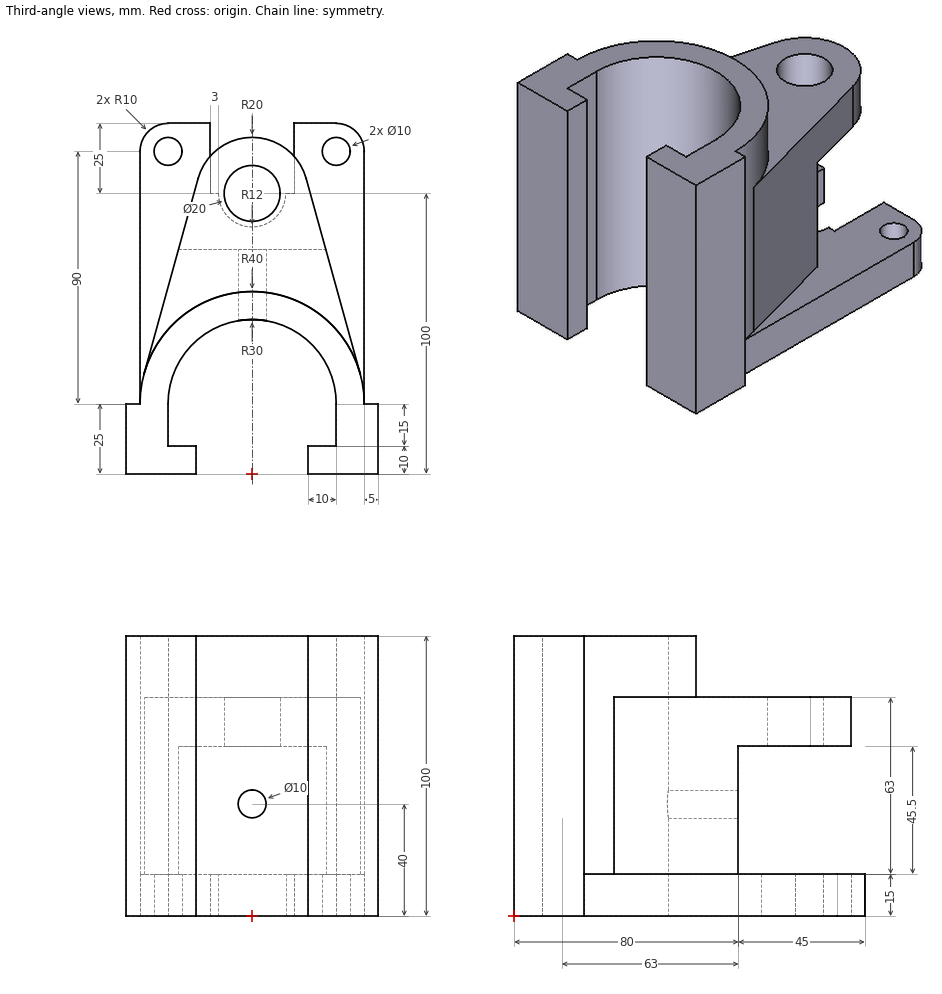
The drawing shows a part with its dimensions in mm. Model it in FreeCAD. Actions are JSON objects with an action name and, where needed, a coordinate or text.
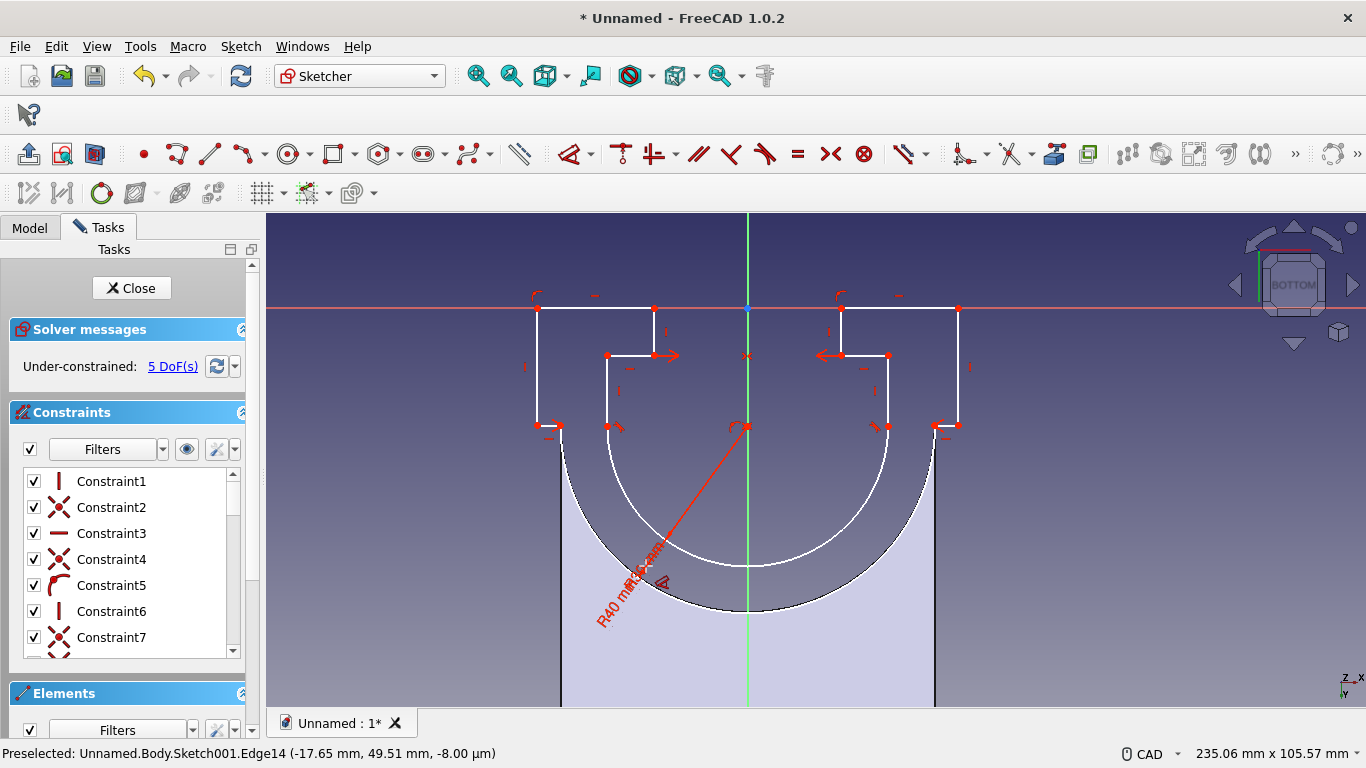
{"action": "scroll", "coordinate": [949, 426], "scroll_direction": "up", "scroll_amount": 3}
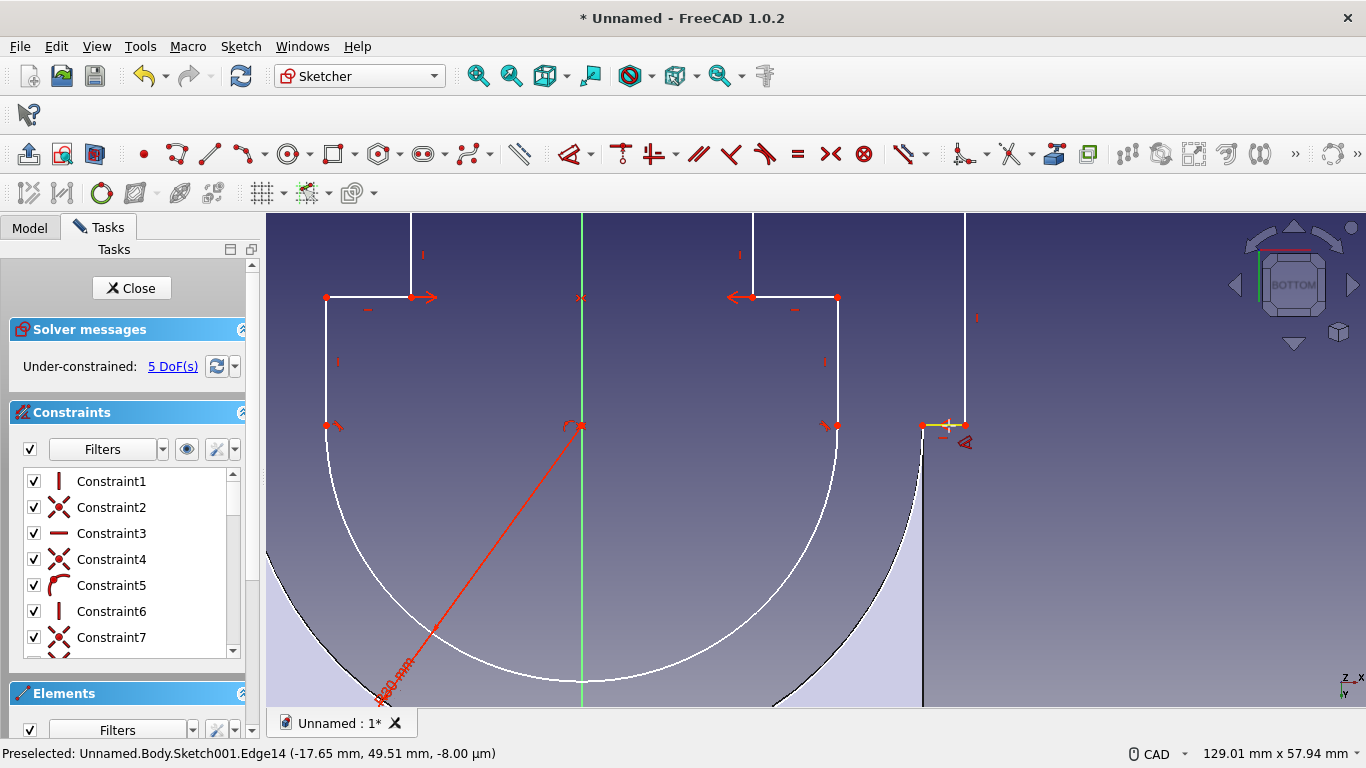
{"action": "left_click", "coordinate": [948, 425]}
{"action": "left_click", "coordinate": [944, 391]}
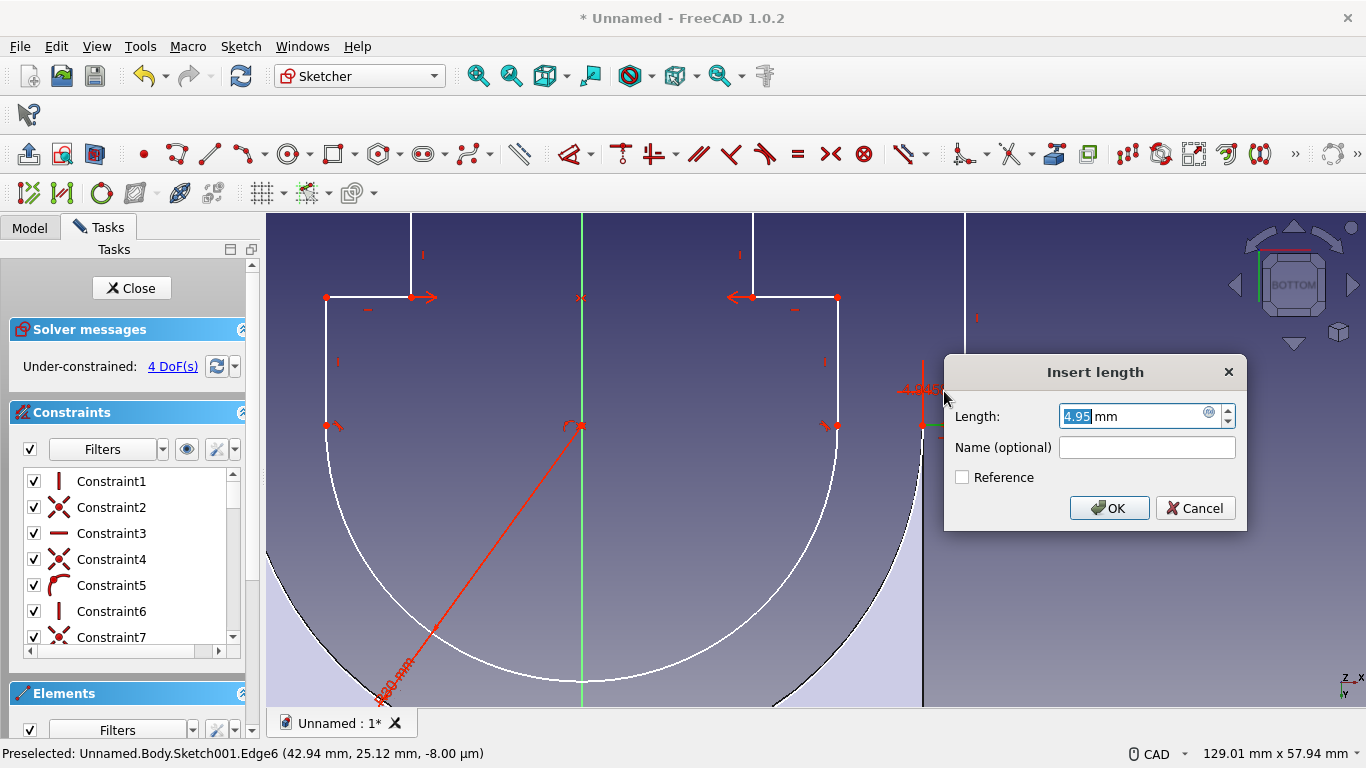
{"action": "type", "text": "5"}
{"action": "key", "text": "Return"}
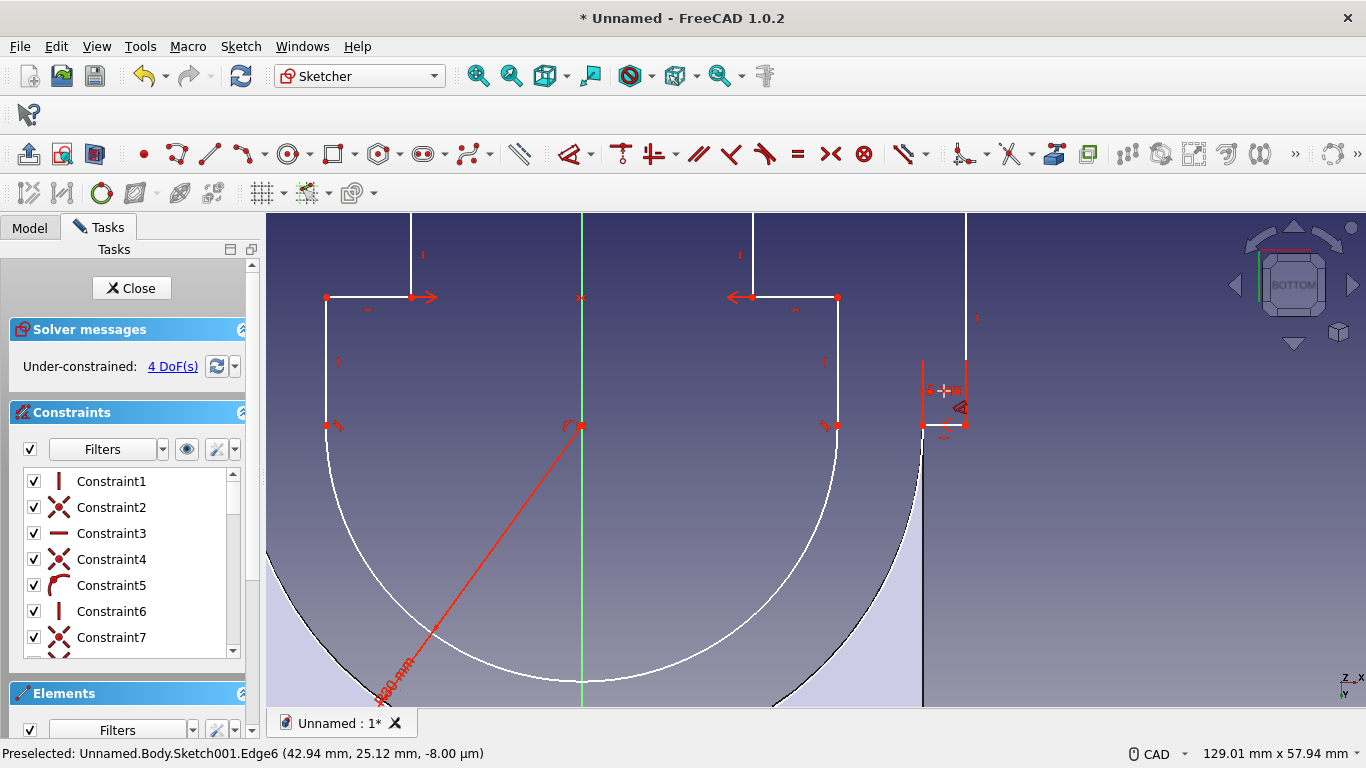
{"action": "left_click", "coordinate": [838, 387]}
{"action": "left_click", "coordinate": [872, 362]}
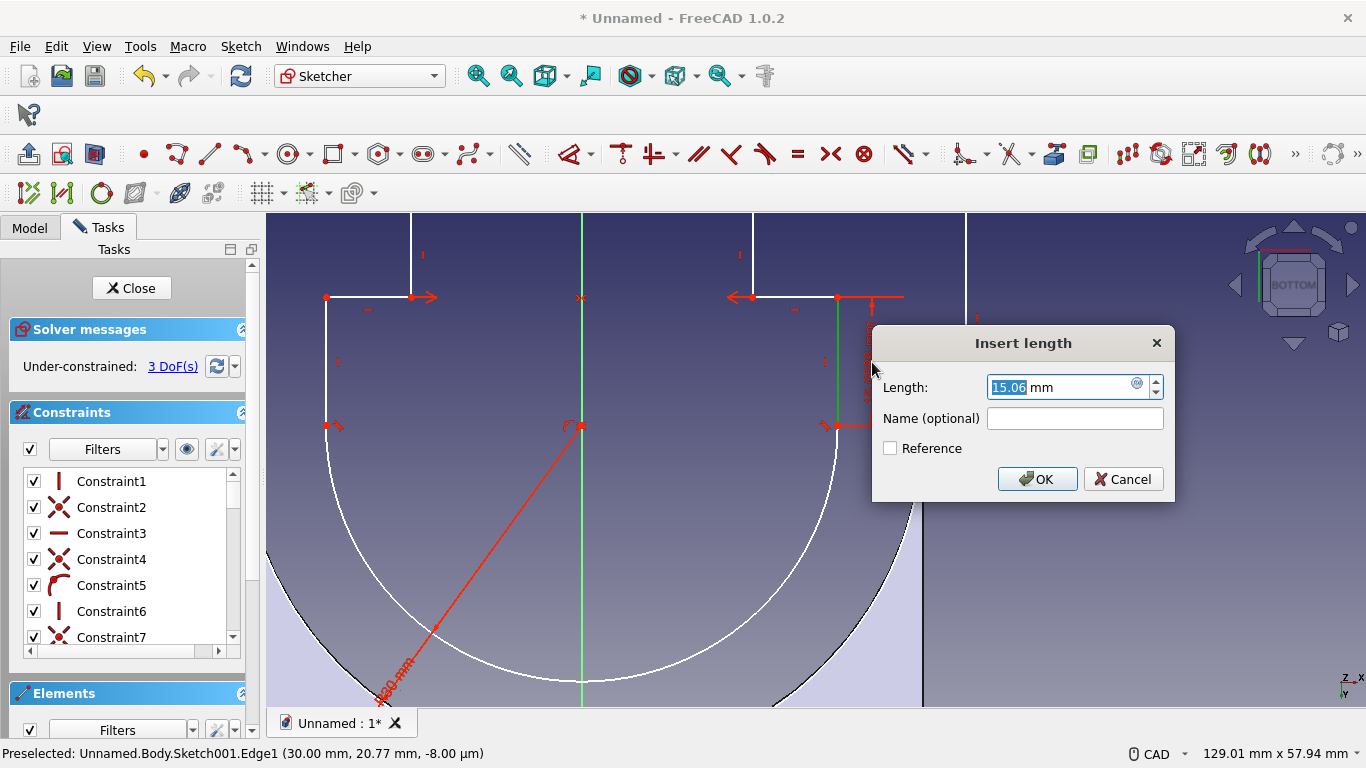
{"action": "type", "text": "15"}
{"action": "key", "text": "Return"}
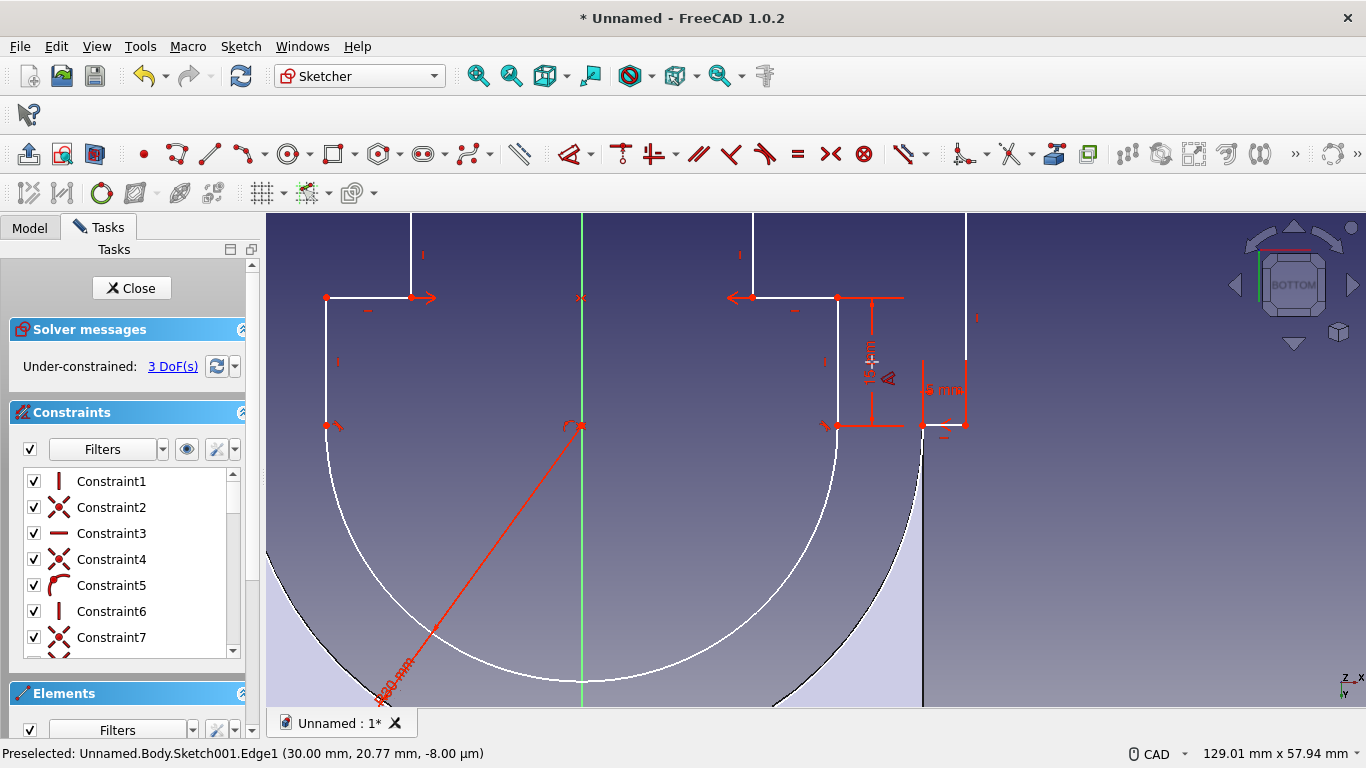
{"action": "left_click", "coordinate": [812, 298]}
{"action": "left_click", "coordinate": [795, 264]}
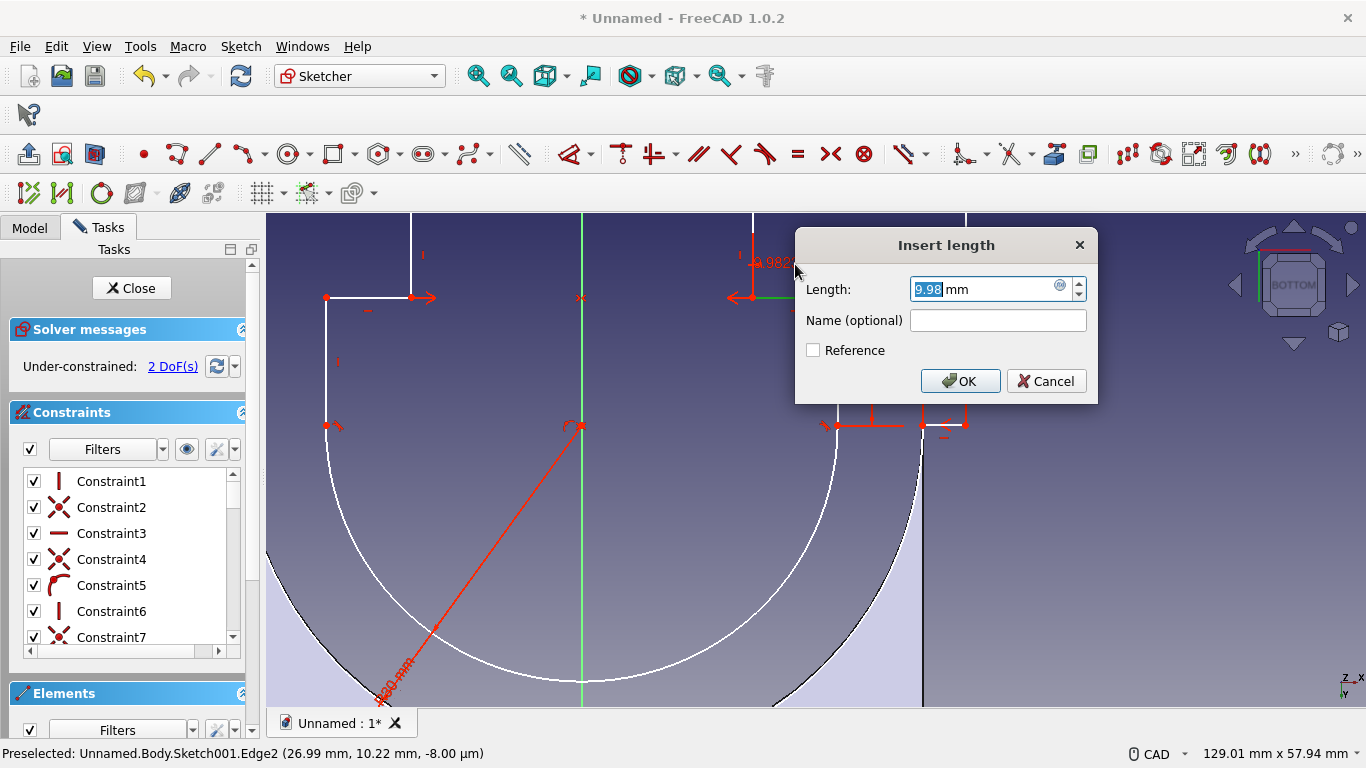
{"action": "type", "text": "10"}
{"action": "key", "text": "Return"}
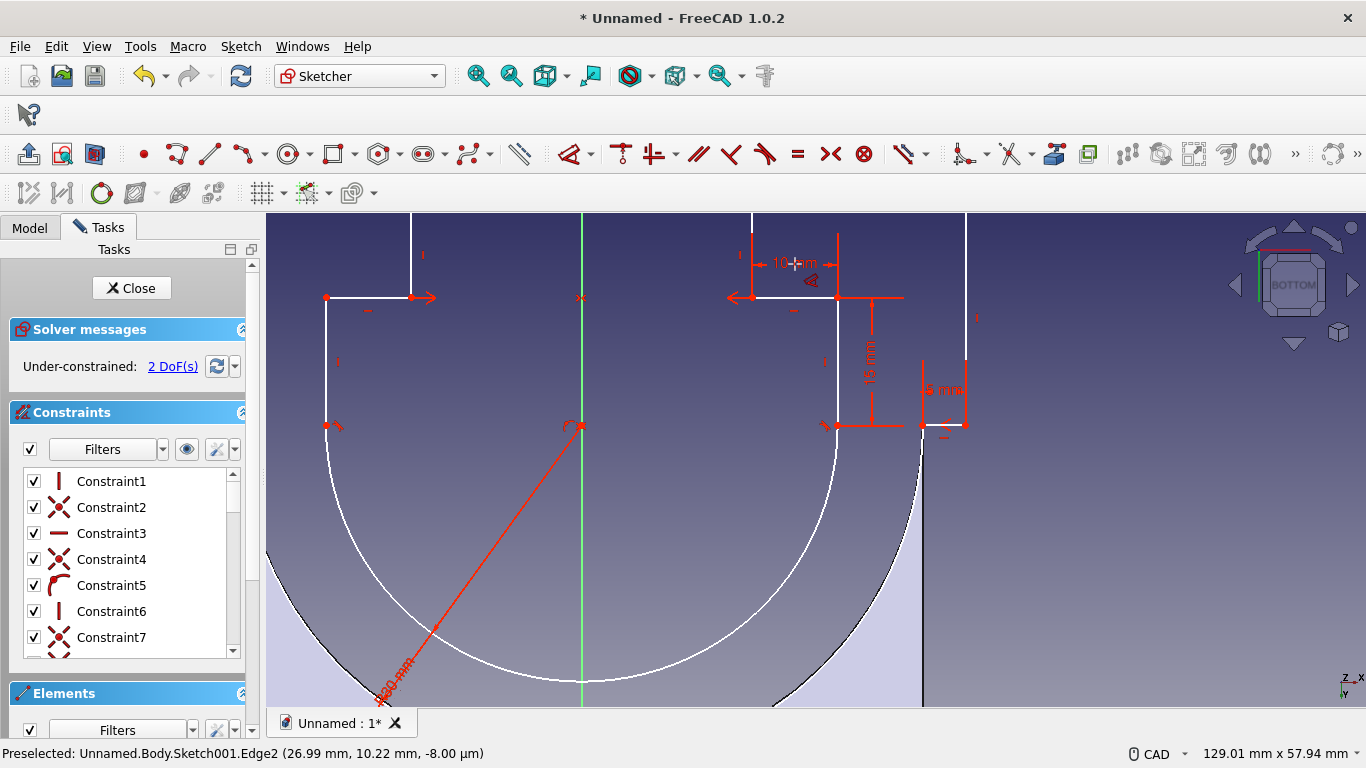
{"action": "left_click", "coordinate": [752, 272]}
{"action": "left_click", "coordinate": [718, 269]}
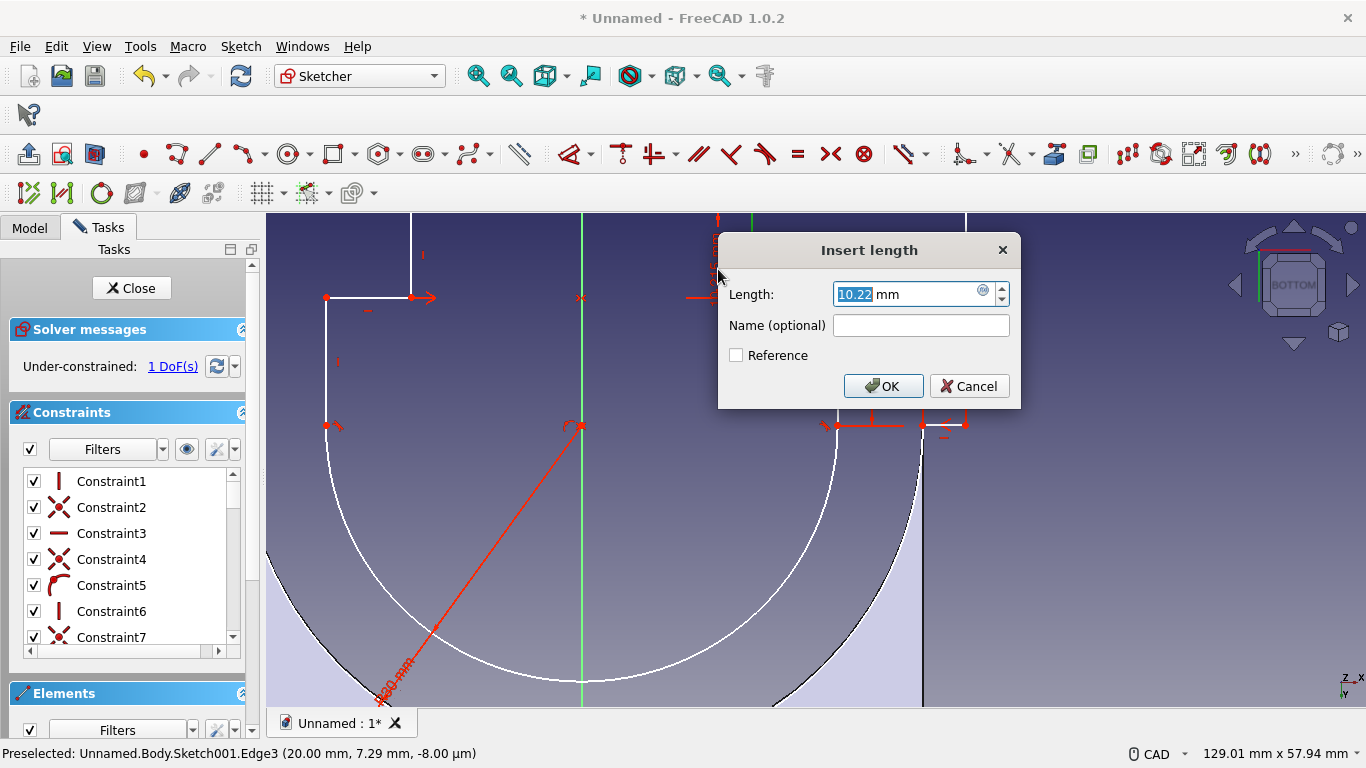
{"action": "type", "text": "10"}
{"action": "key", "text": "Return"}